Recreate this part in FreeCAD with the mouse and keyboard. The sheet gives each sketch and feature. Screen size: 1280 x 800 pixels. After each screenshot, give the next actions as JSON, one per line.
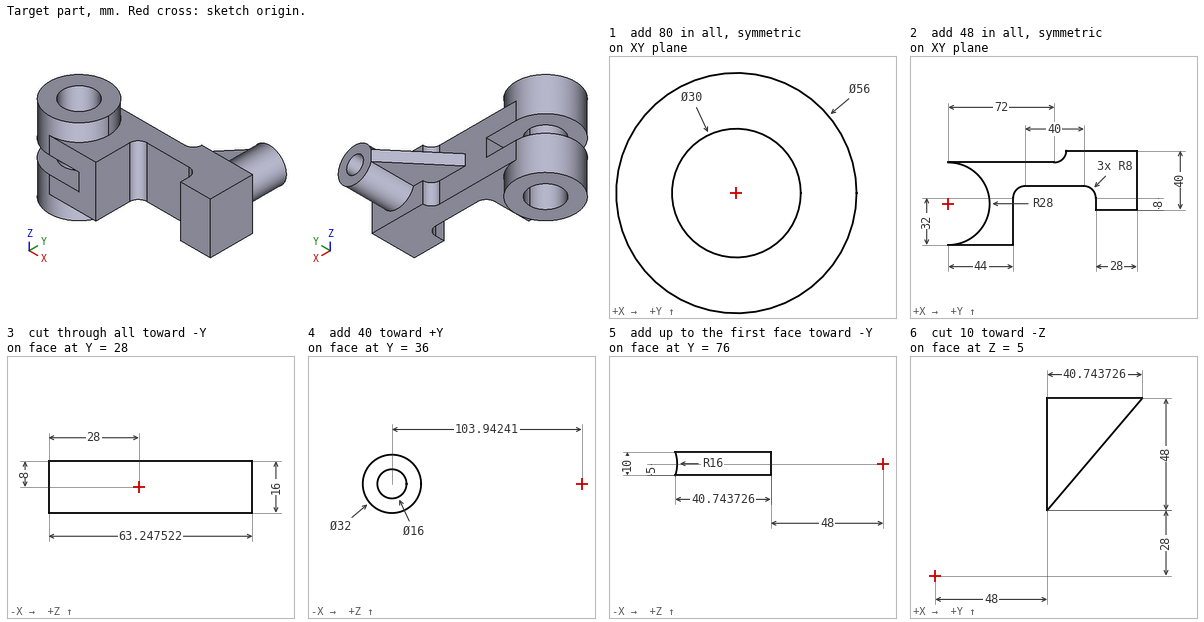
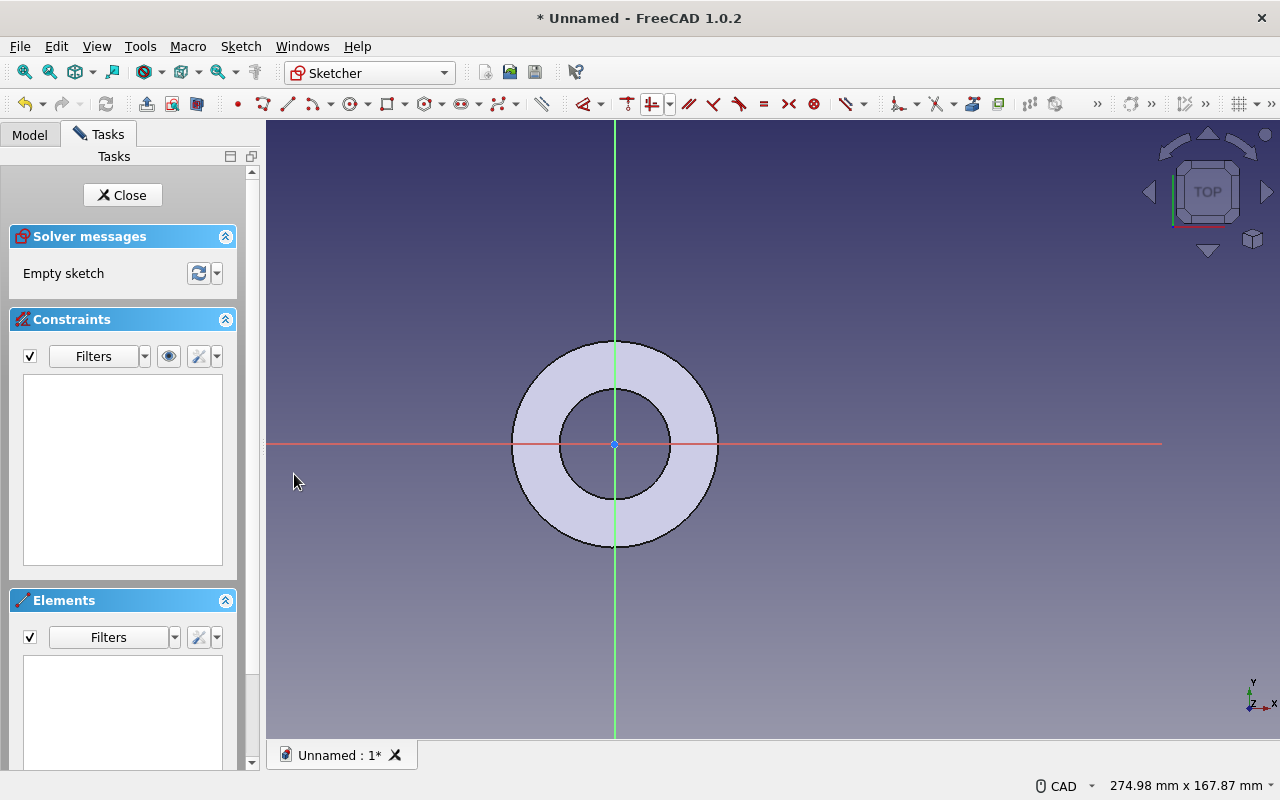
{"action": "key", "text": "g l"}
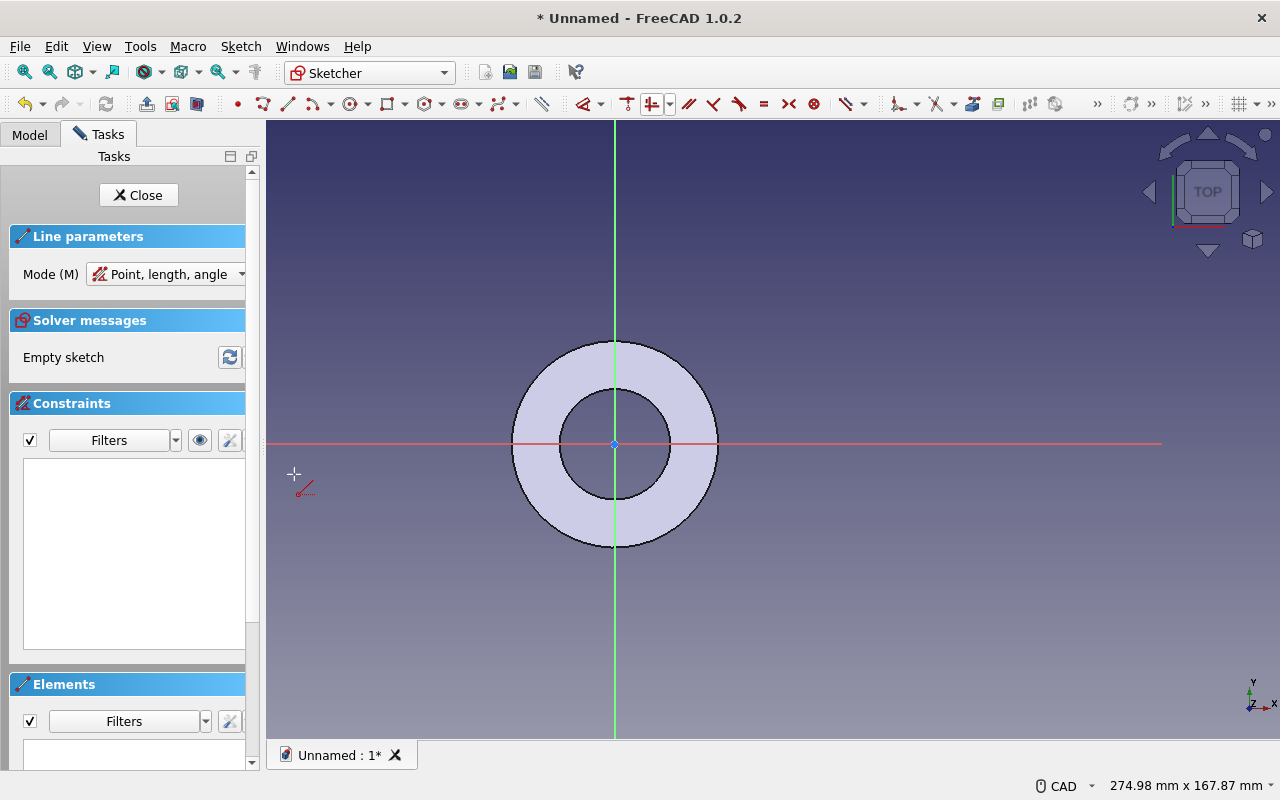
{"action": "left_click", "coordinate": [880, 341]}
{"action": "left_click", "coordinate": [615, 341]}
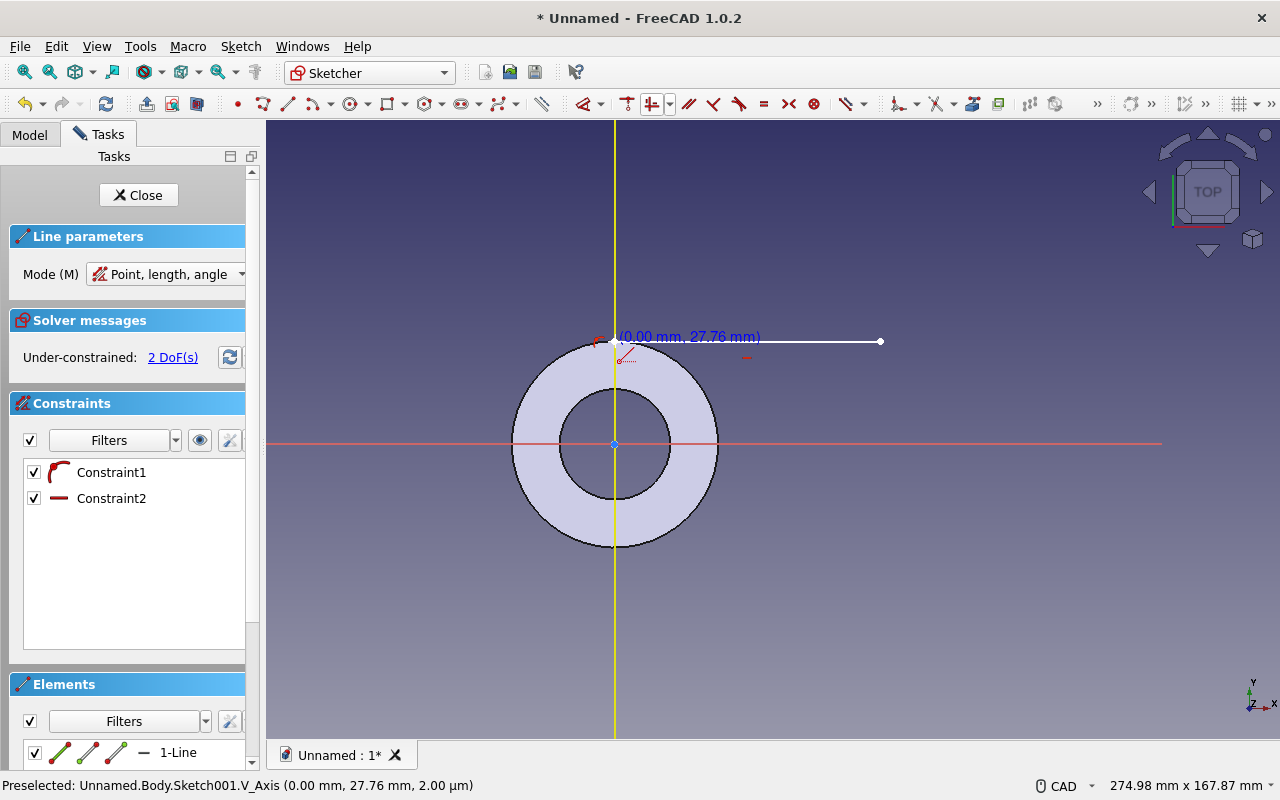
{"action": "left_click", "coordinate": [263, 104]}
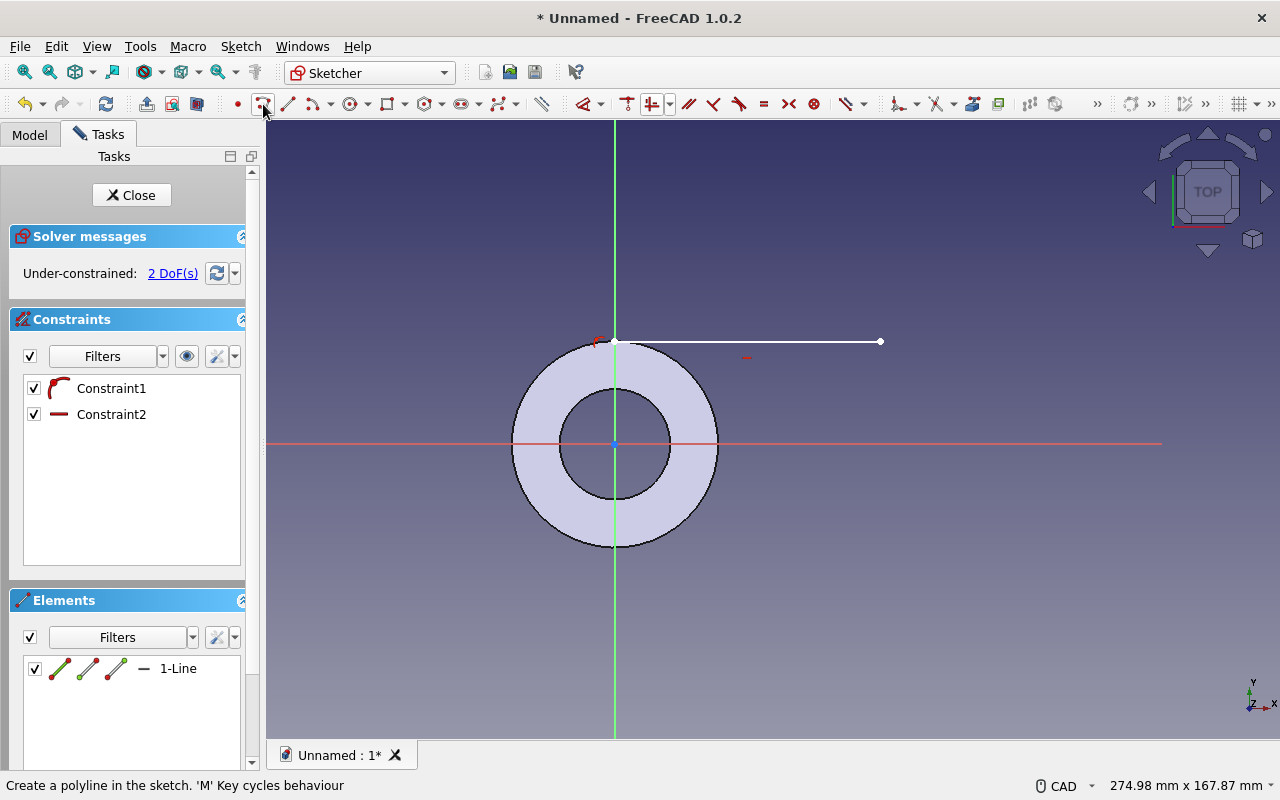
{"action": "left_click", "coordinate": [615, 548]}
{"action": "left_click", "coordinate": [777, 548]}
{"action": "left_click", "coordinate": [777, 430]}
{"action": "right_click", "coordinate": [777, 430]}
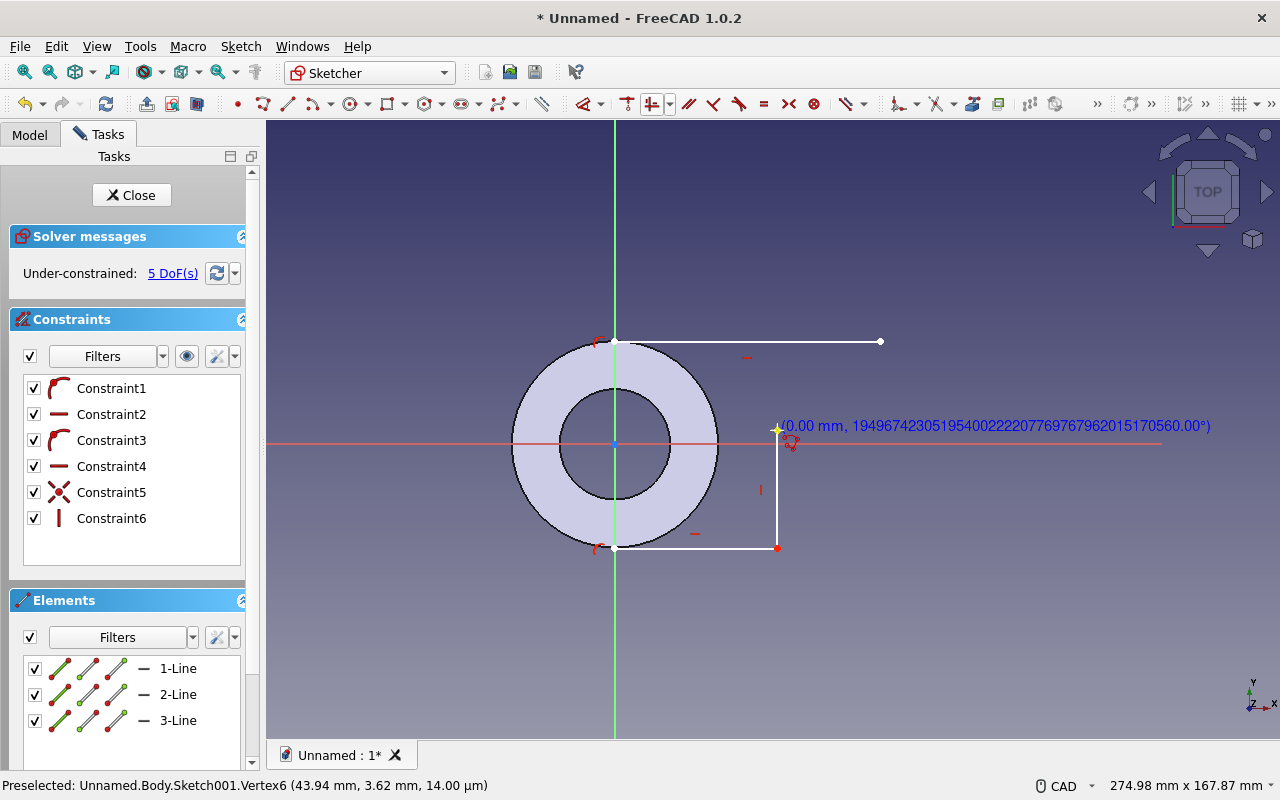
{"action": "key", "text": "g l"}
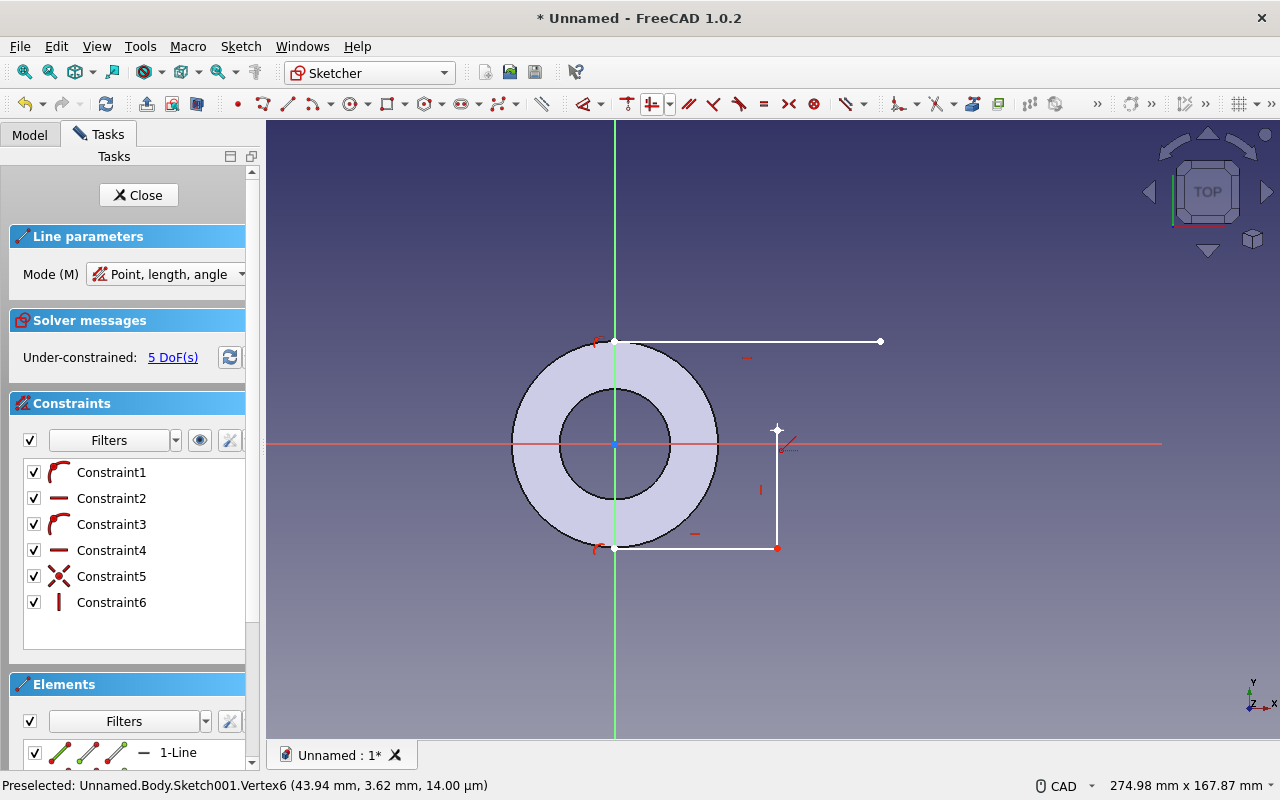
{"action": "left_click", "coordinate": [807, 400]}
{"action": "left_click", "coordinate": [954, 400]}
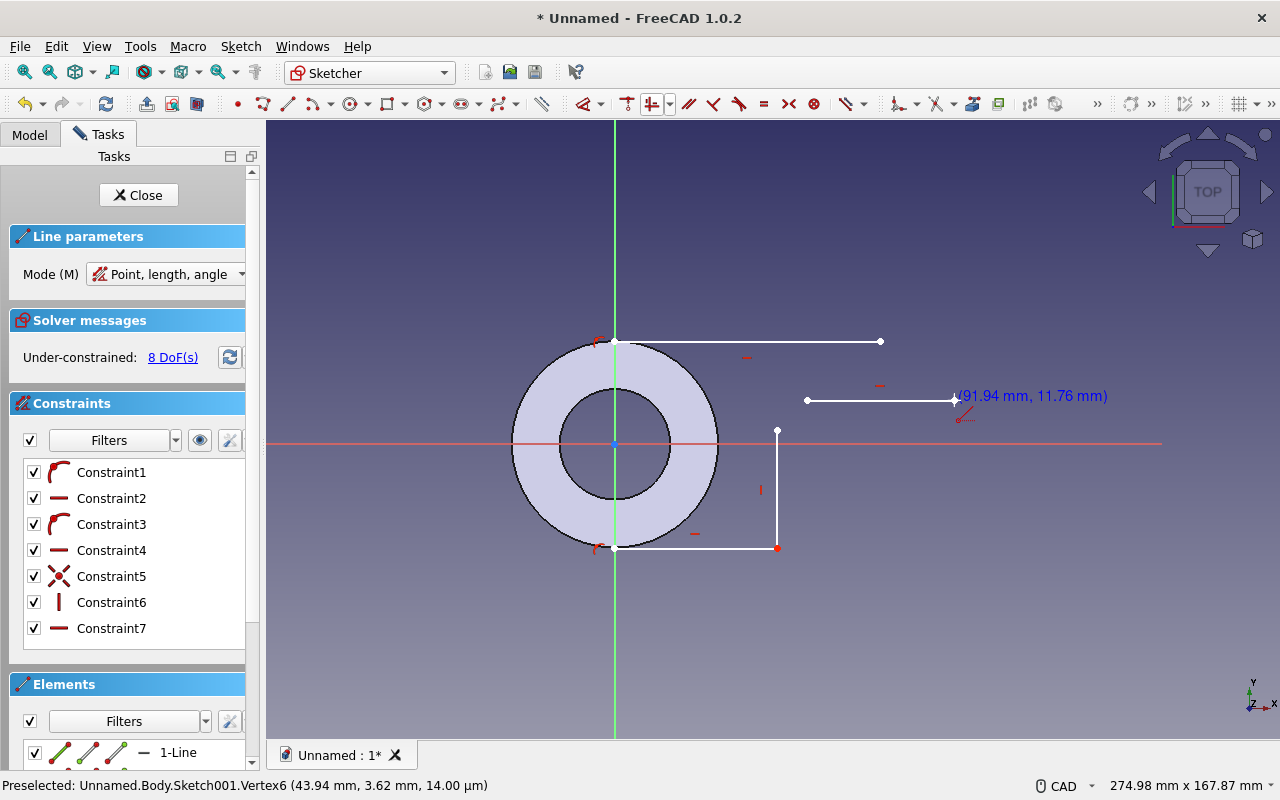
{"action": "left_click", "coordinate": [263, 104]}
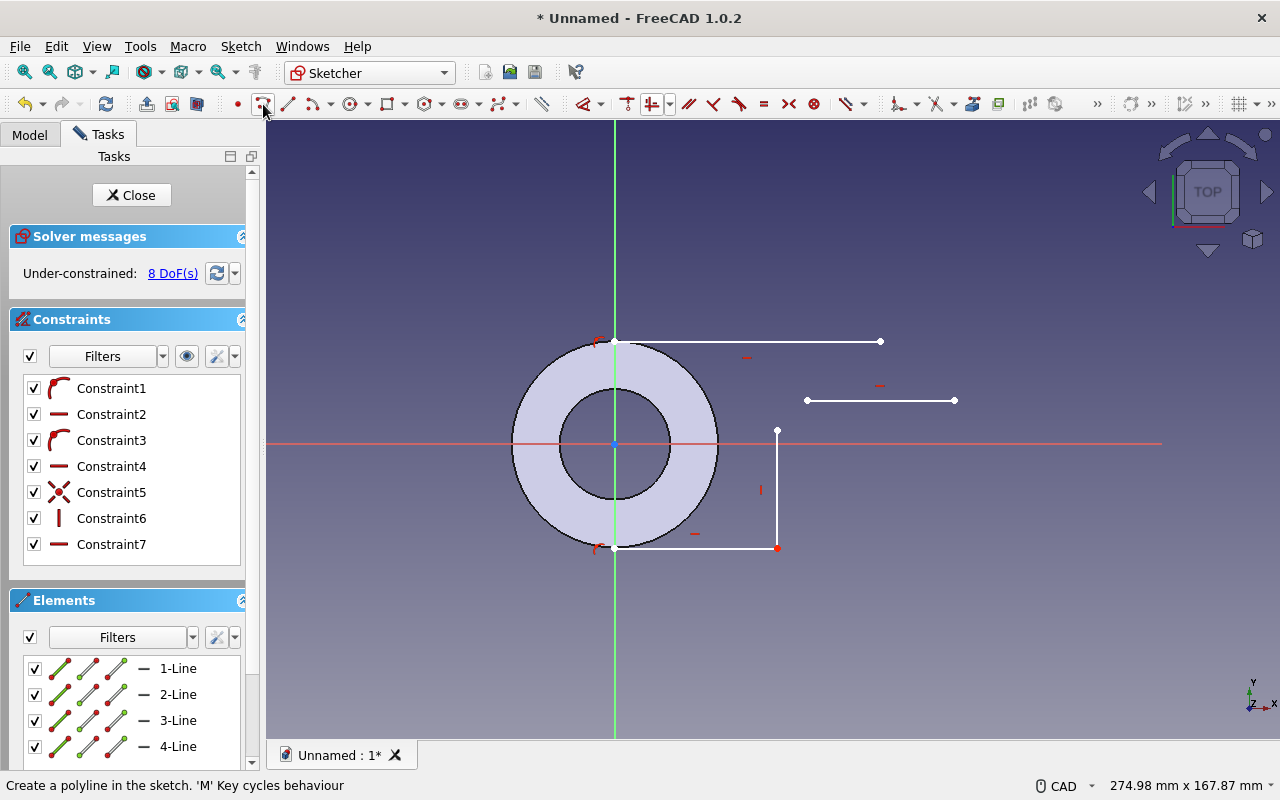
{"action": "left_click", "coordinate": [984, 430]}
{"action": "left_click", "coordinate": [984, 459]}
{"action": "left_click", "coordinate": [1087, 459]}
{"action": "left_click", "coordinate": [1087, 312]}
{"action": "left_click", "coordinate": [910, 312]}
{"action": "right_click", "coordinate": [910, 312]}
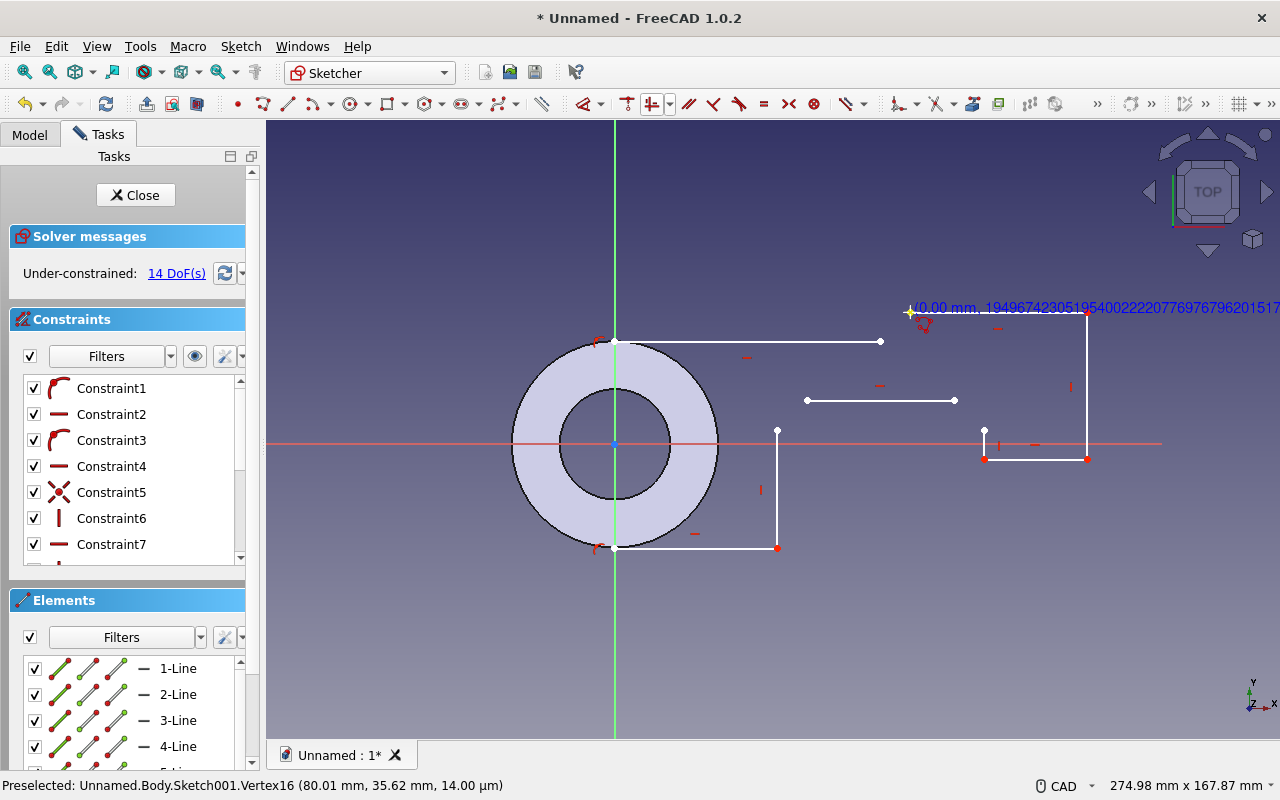
{"action": "key", "text": "g 3 a"}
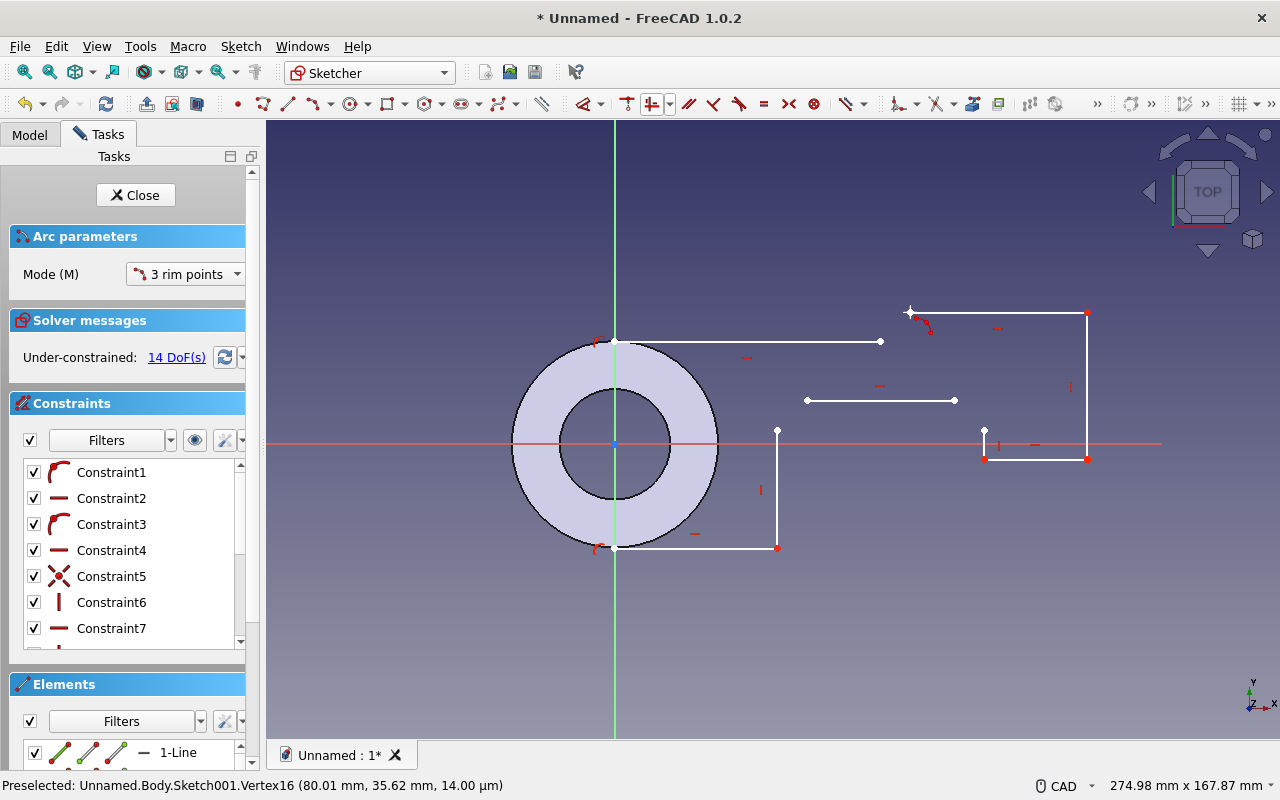
{"action": "left_click", "coordinate": [615, 342]}
{"action": "left_click", "coordinate": [615, 549]}
{"action": "left_click", "coordinate": [713, 476]}